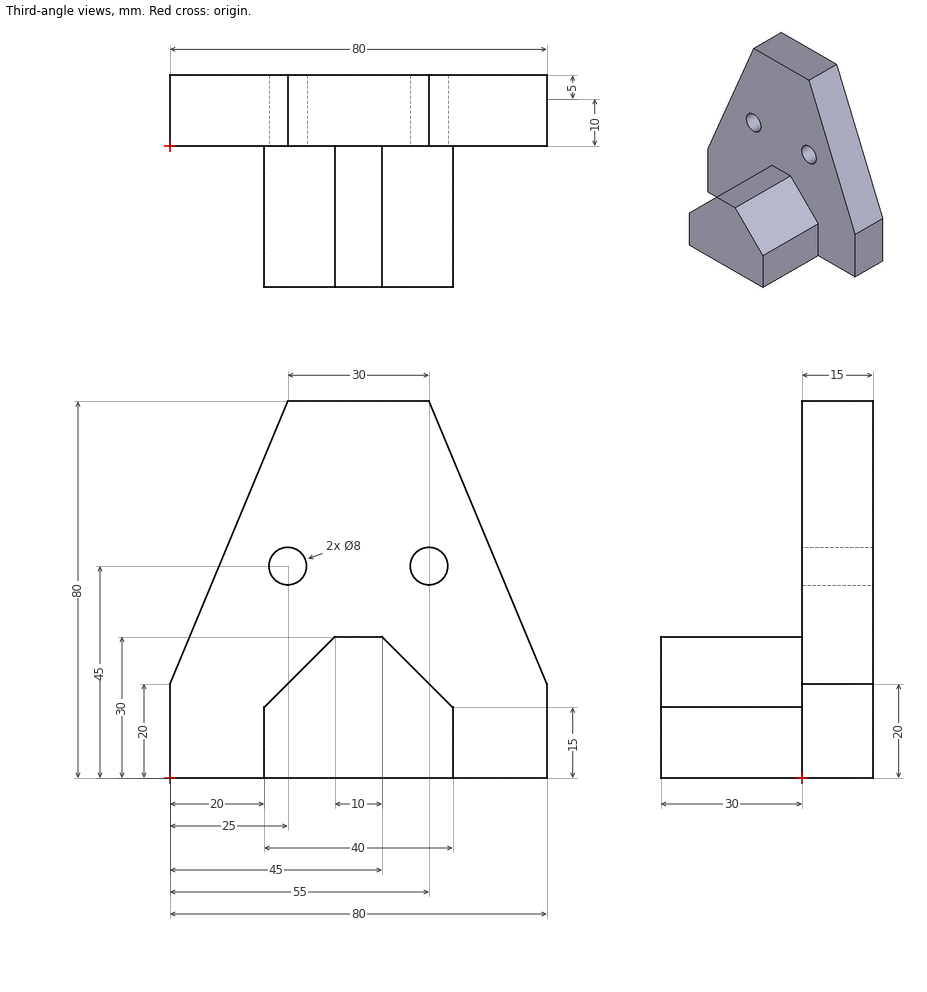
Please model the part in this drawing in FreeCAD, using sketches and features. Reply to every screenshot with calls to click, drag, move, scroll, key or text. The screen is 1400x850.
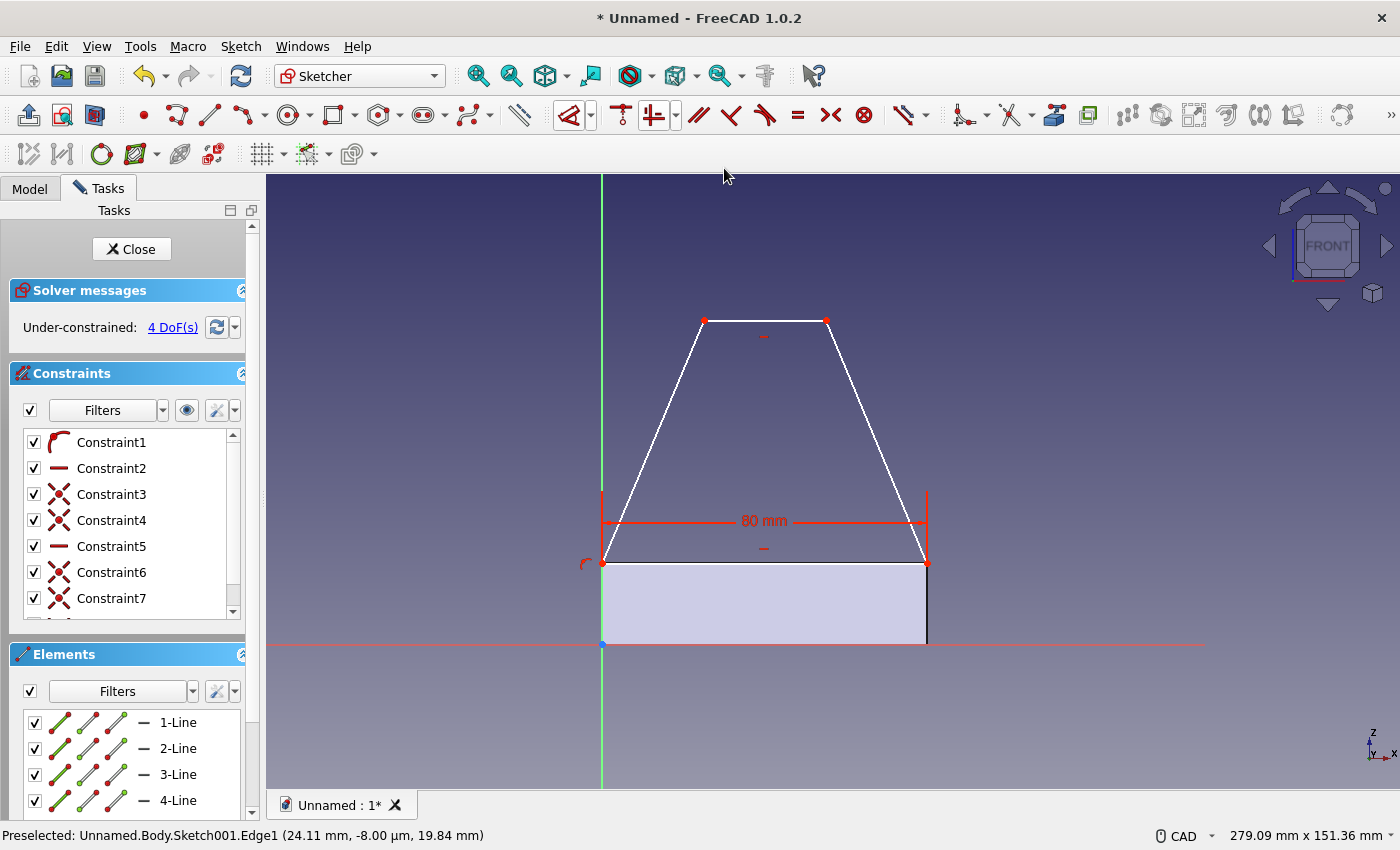
click(789, 321)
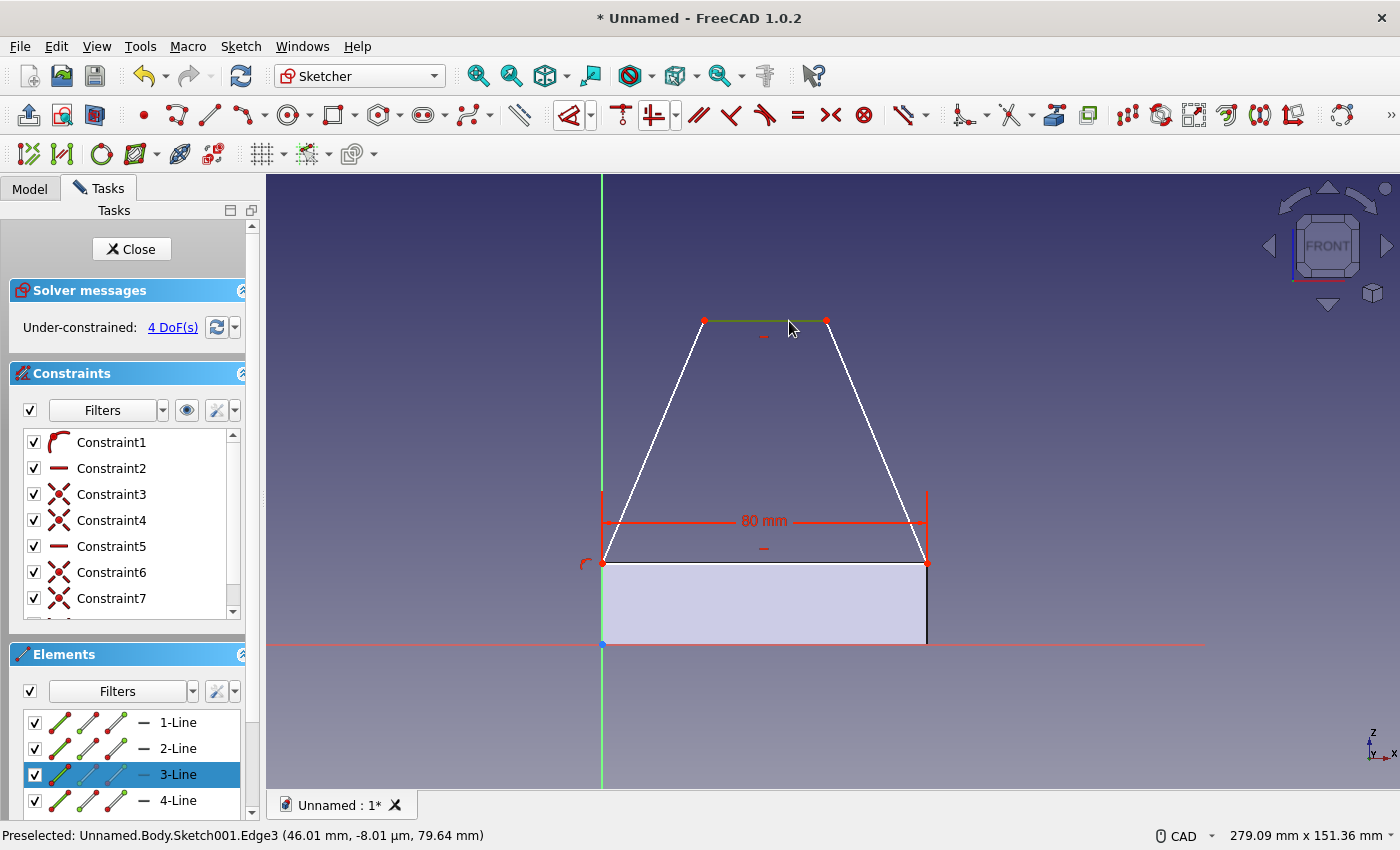
key(l)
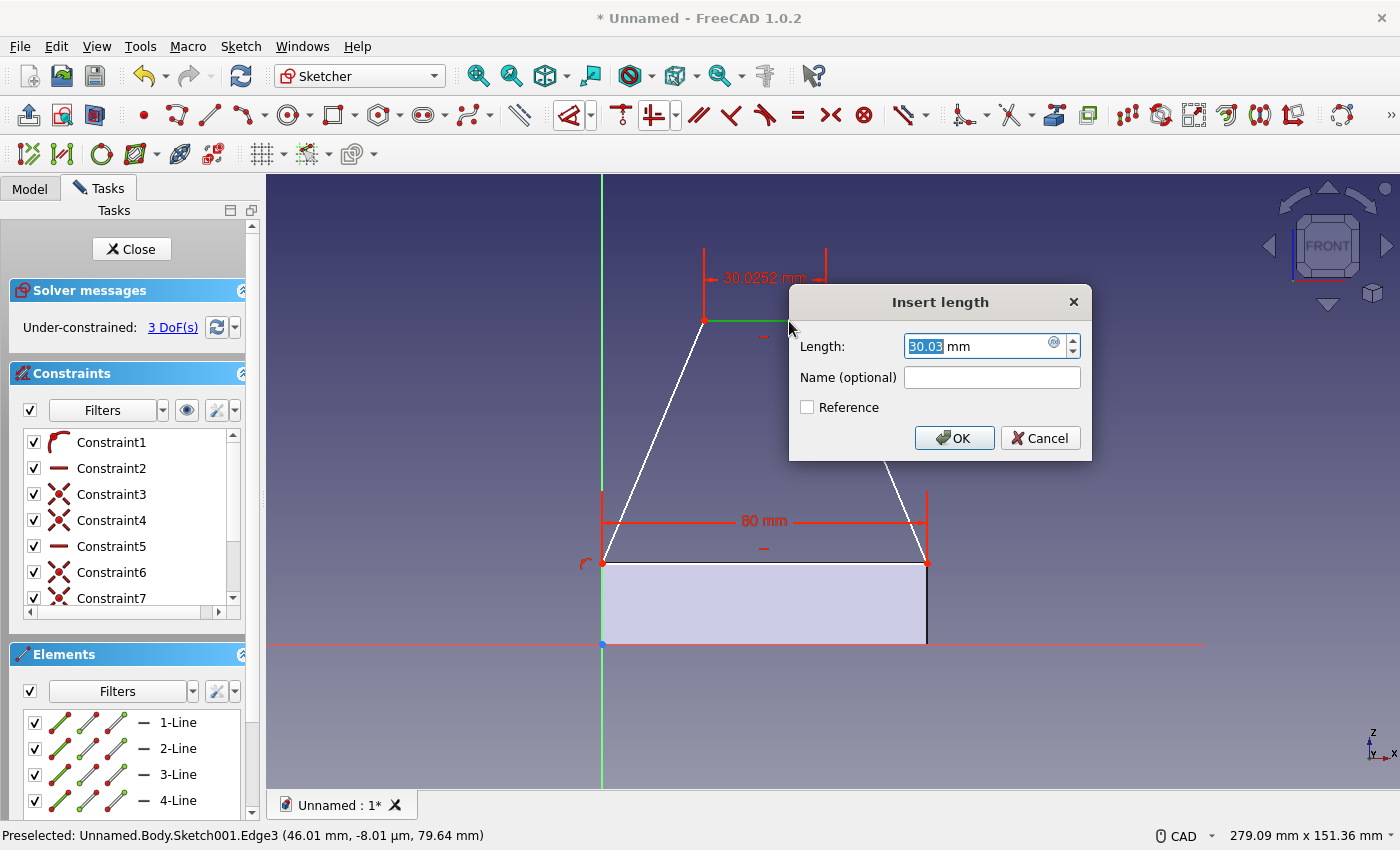
text(30)
key(Return)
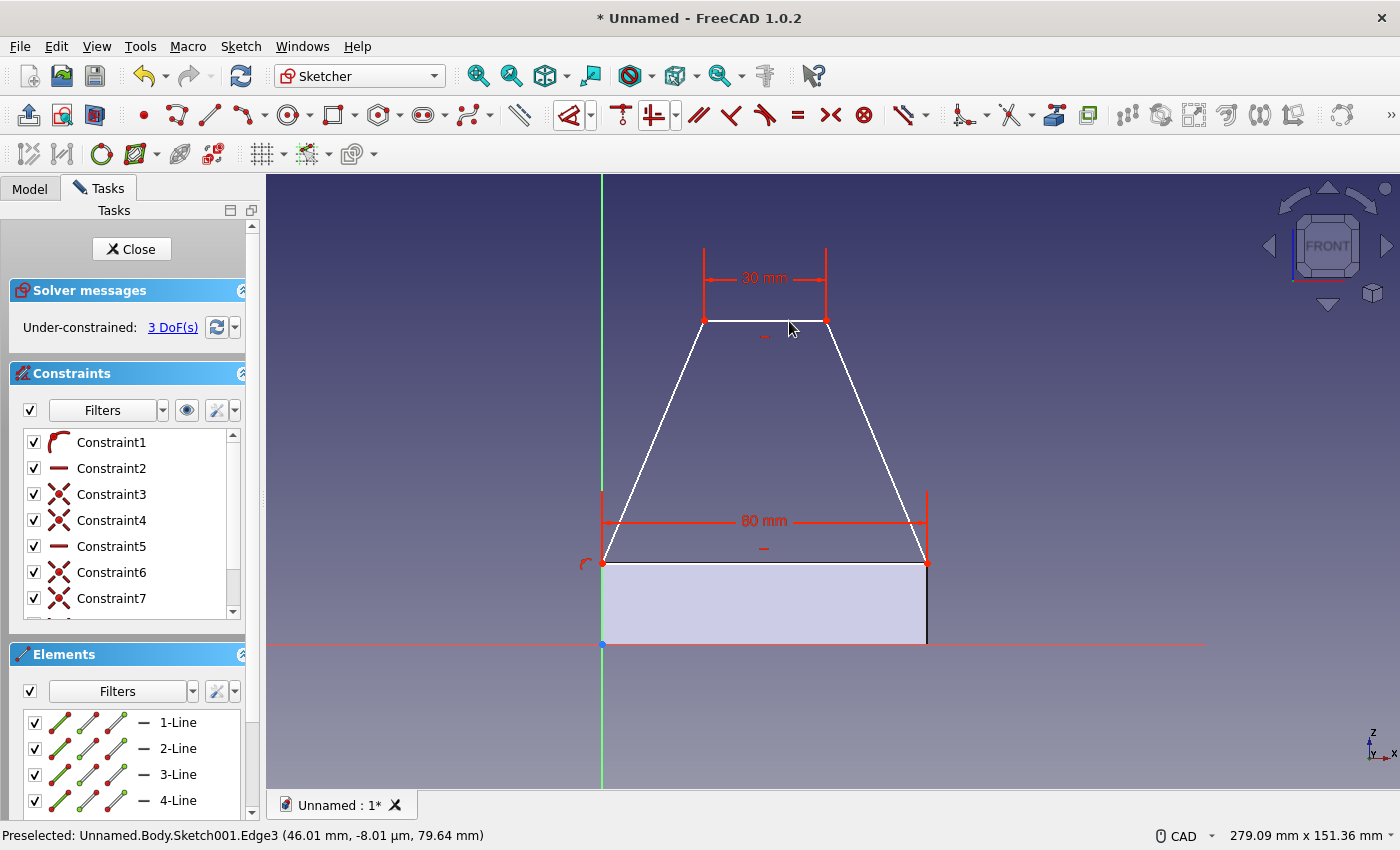
click(602, 564)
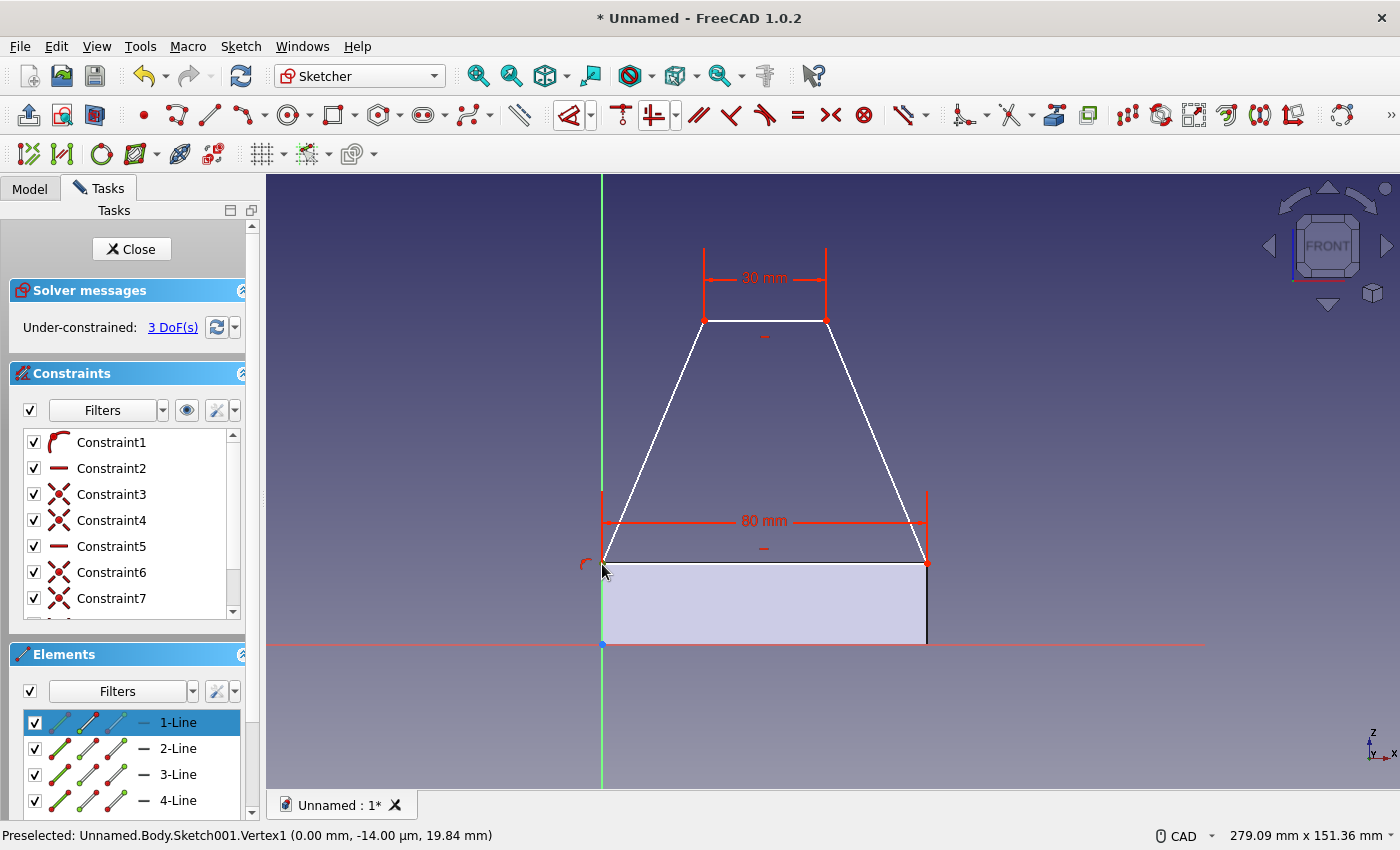
click(590, 116)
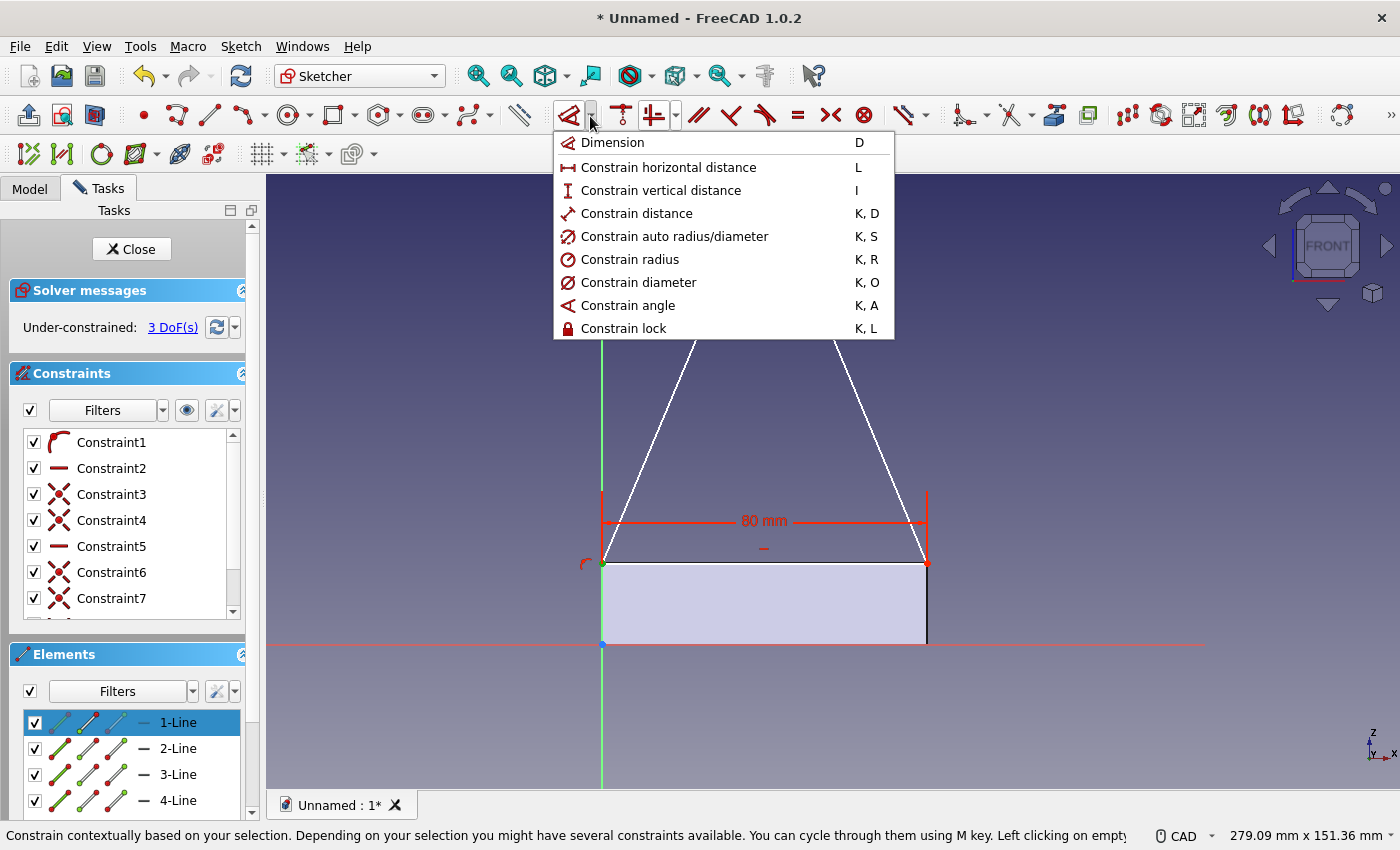
click(724, 190)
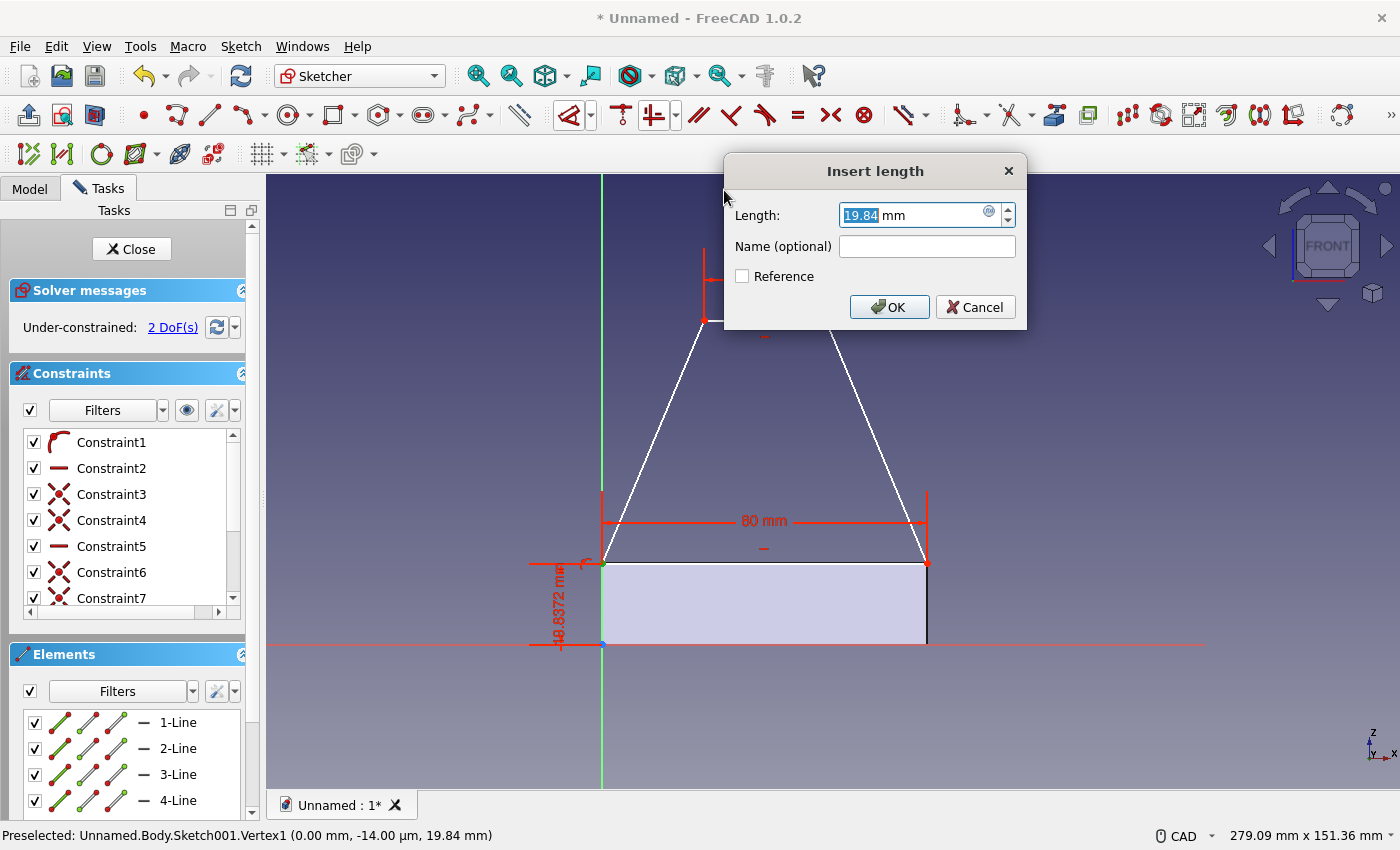
text(20)
key(Return)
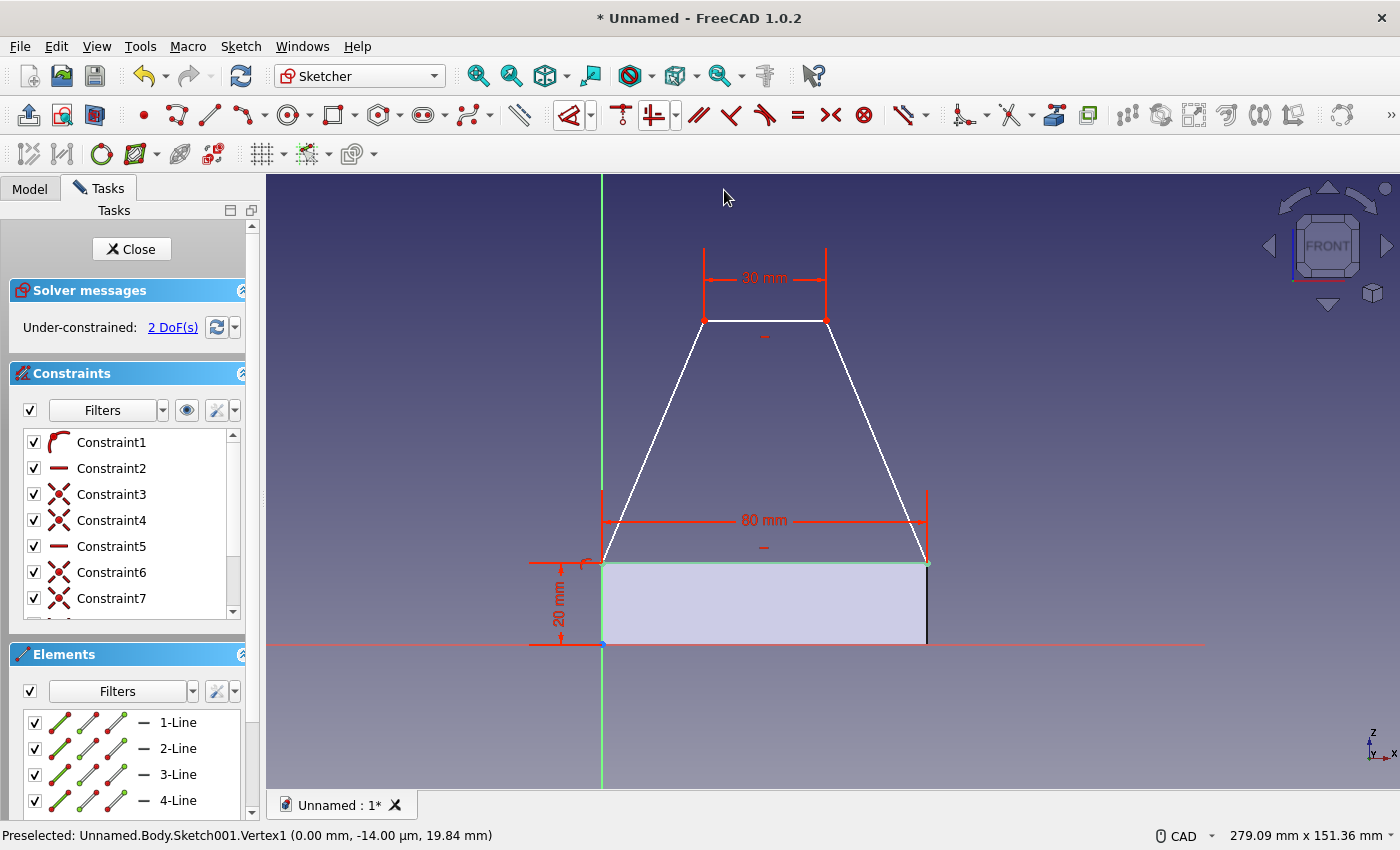
click(826, 321)